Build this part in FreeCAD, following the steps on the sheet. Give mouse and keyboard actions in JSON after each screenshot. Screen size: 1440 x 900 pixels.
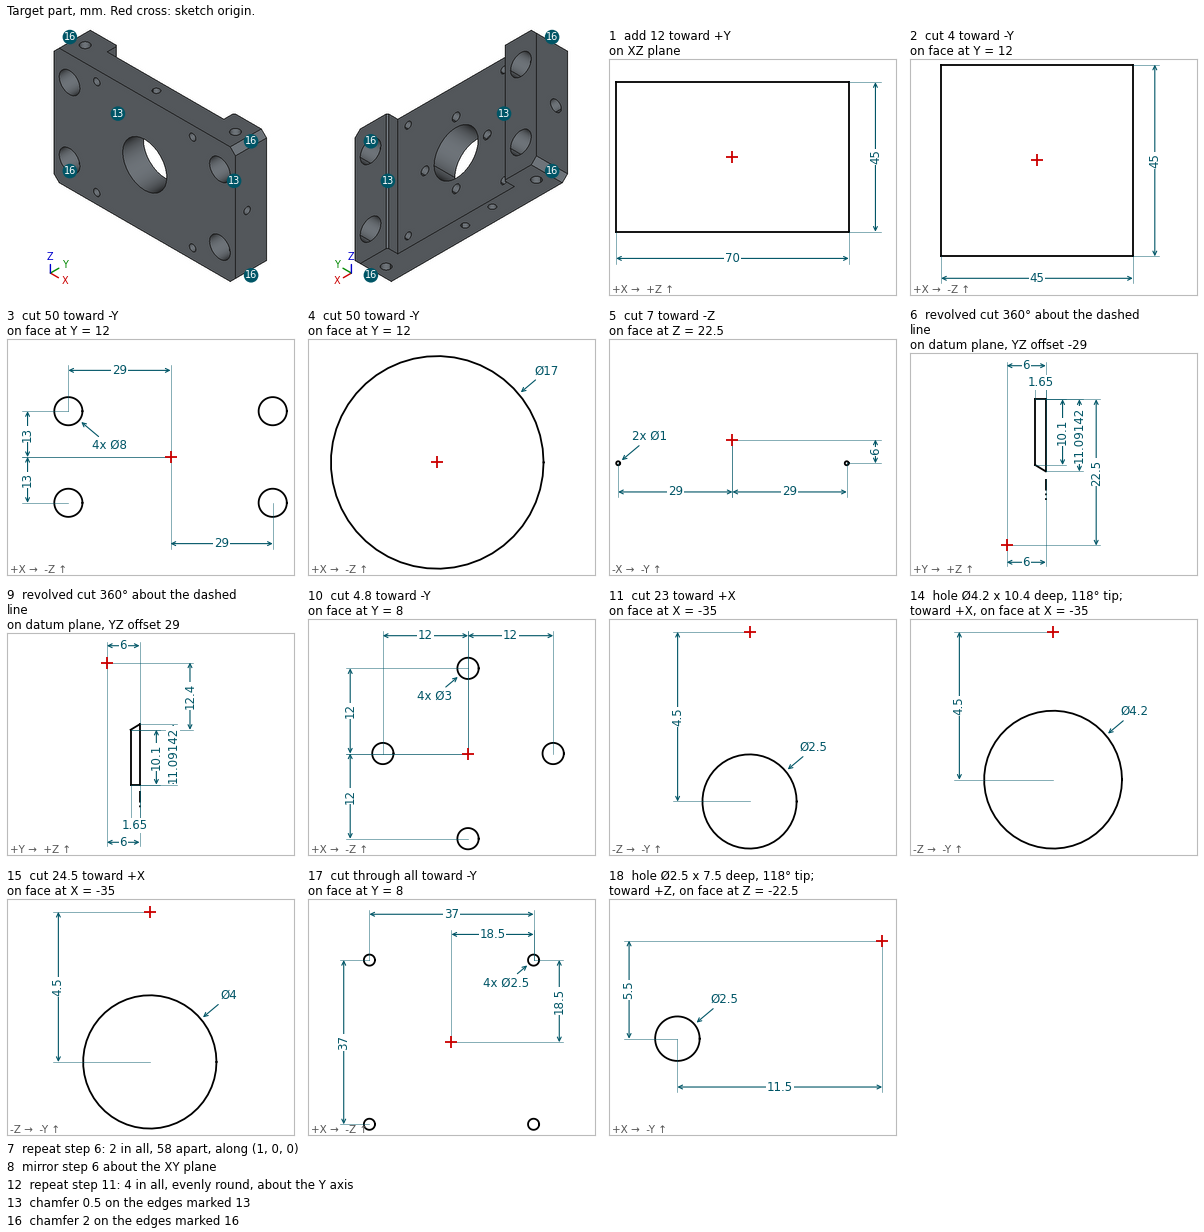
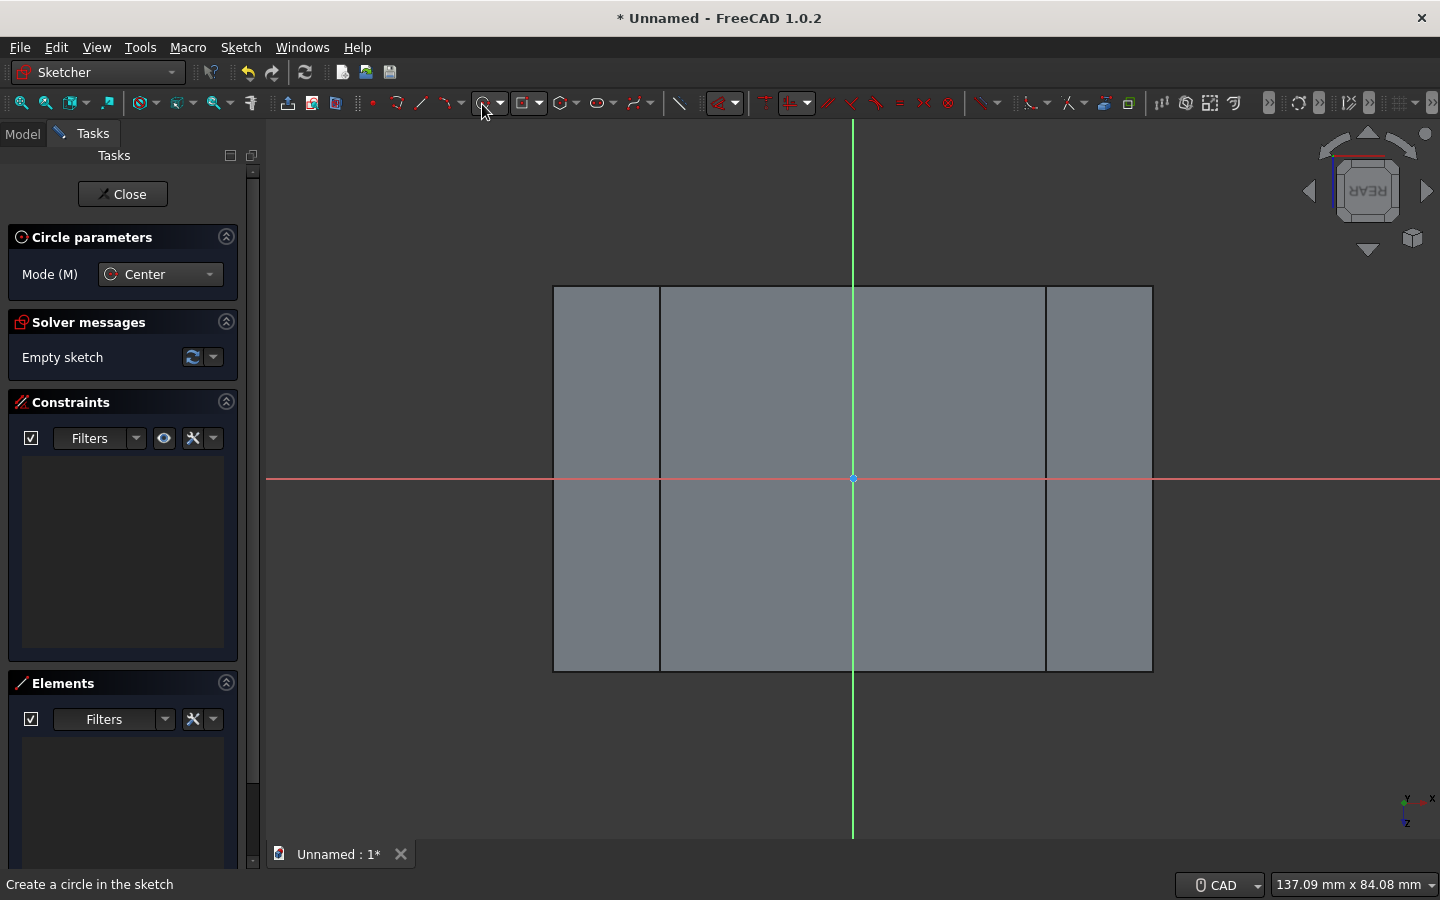
{"action": "left_click", "coordinate": [605, 368]}
{"action": "mouse_move", "coordinate": [629, 343]}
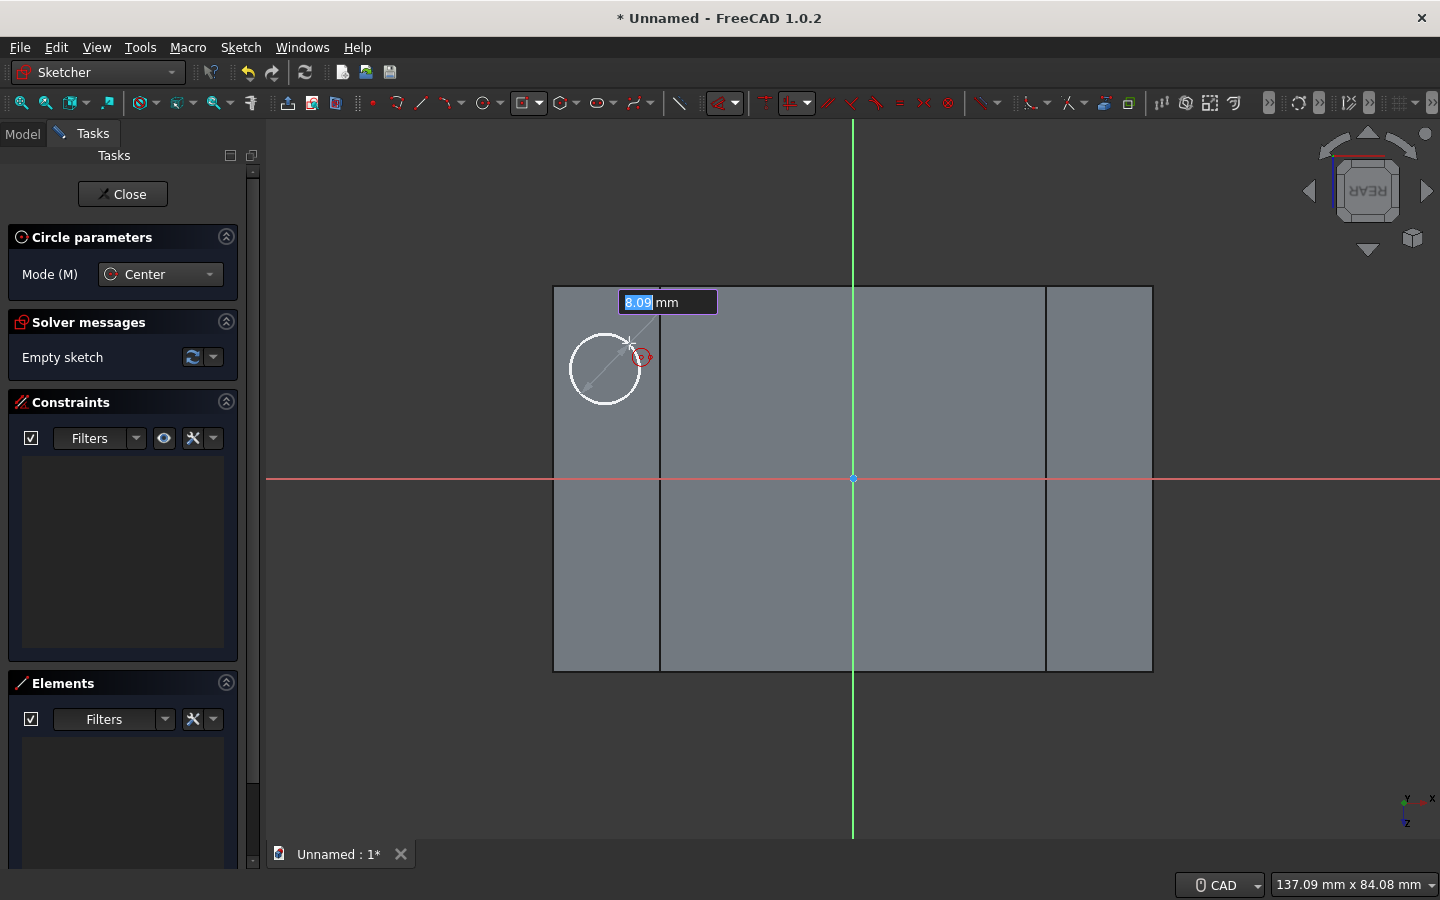
{"action": "type", "text": "8"}
{"action": "key", "text": "Return"}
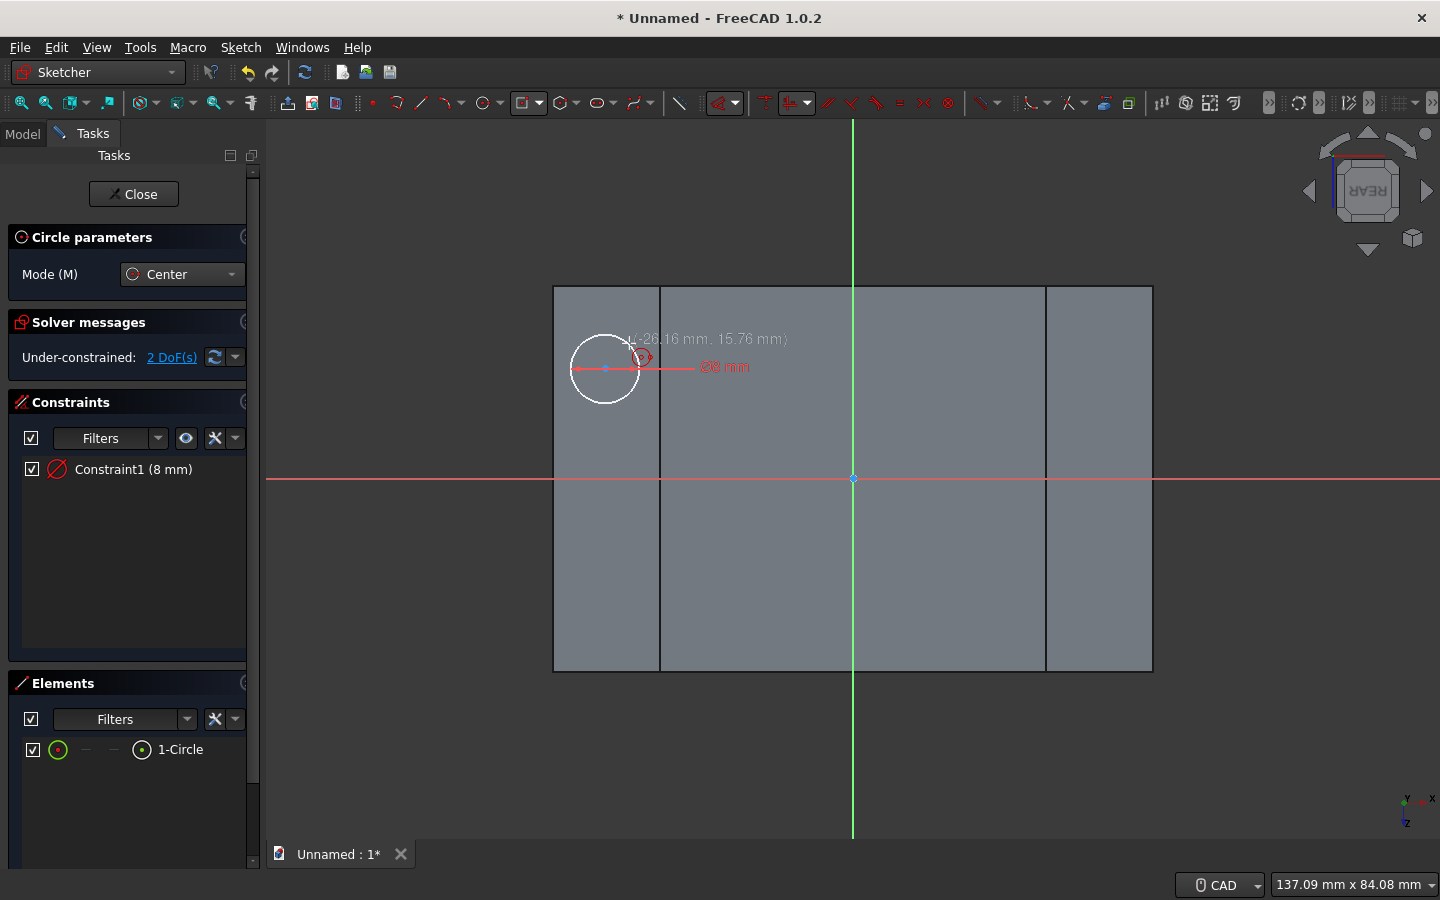
{"action": "left_click", "coordinate": [605, 590]}
{"action": "mouse_move", "coordinate": [629, 566]}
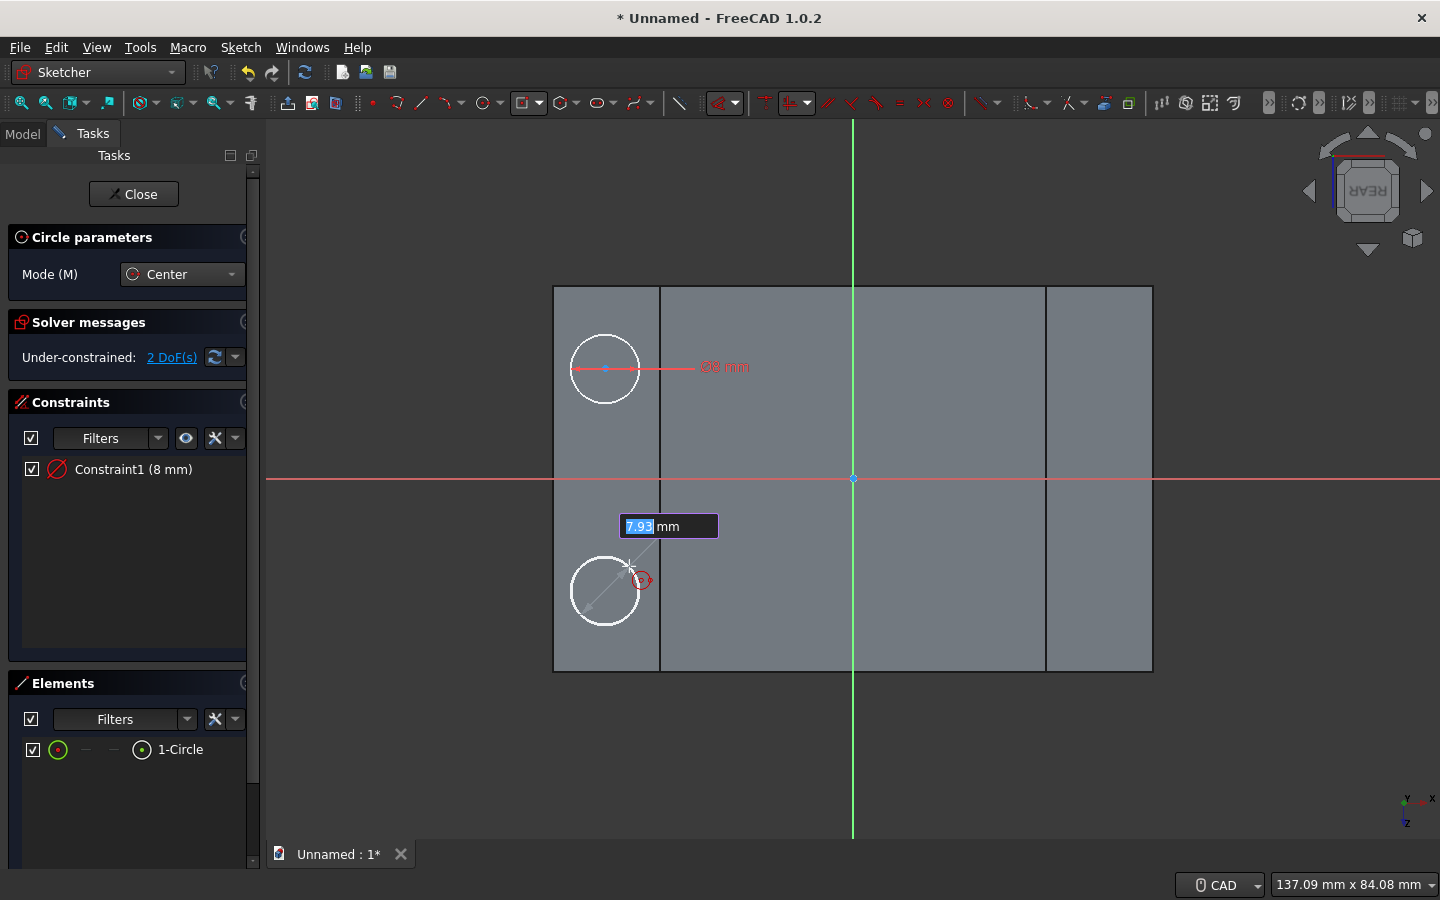
{"action": "type", "text": "8"}
{"action": "key", "text": "Return"}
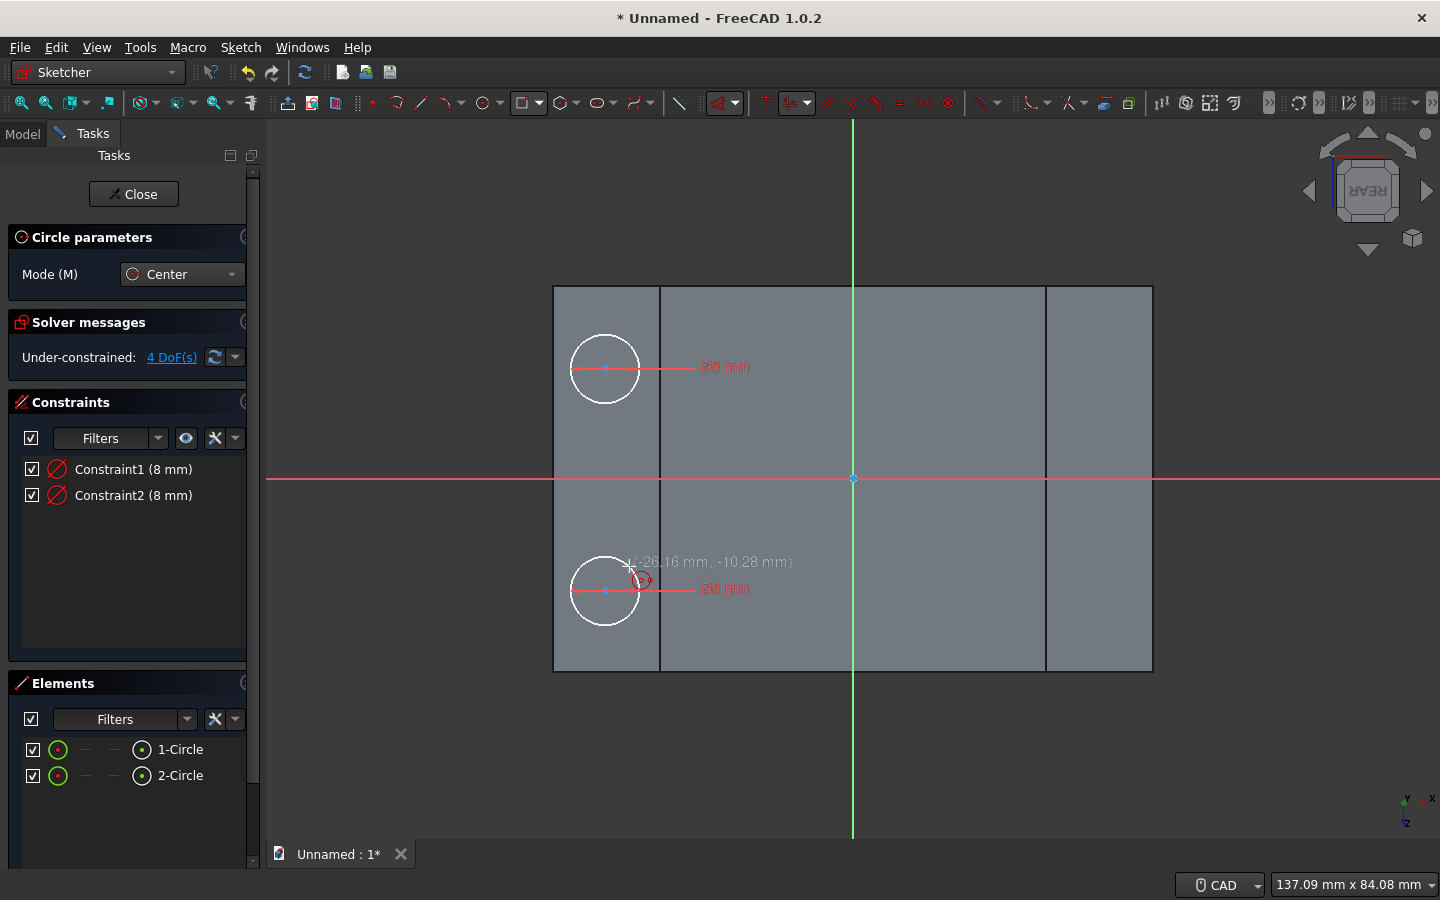
{"action": "left_click", "coordinate": [1101, 590]}
{"action": "mouse_move", "coordinate": [1126, 566]}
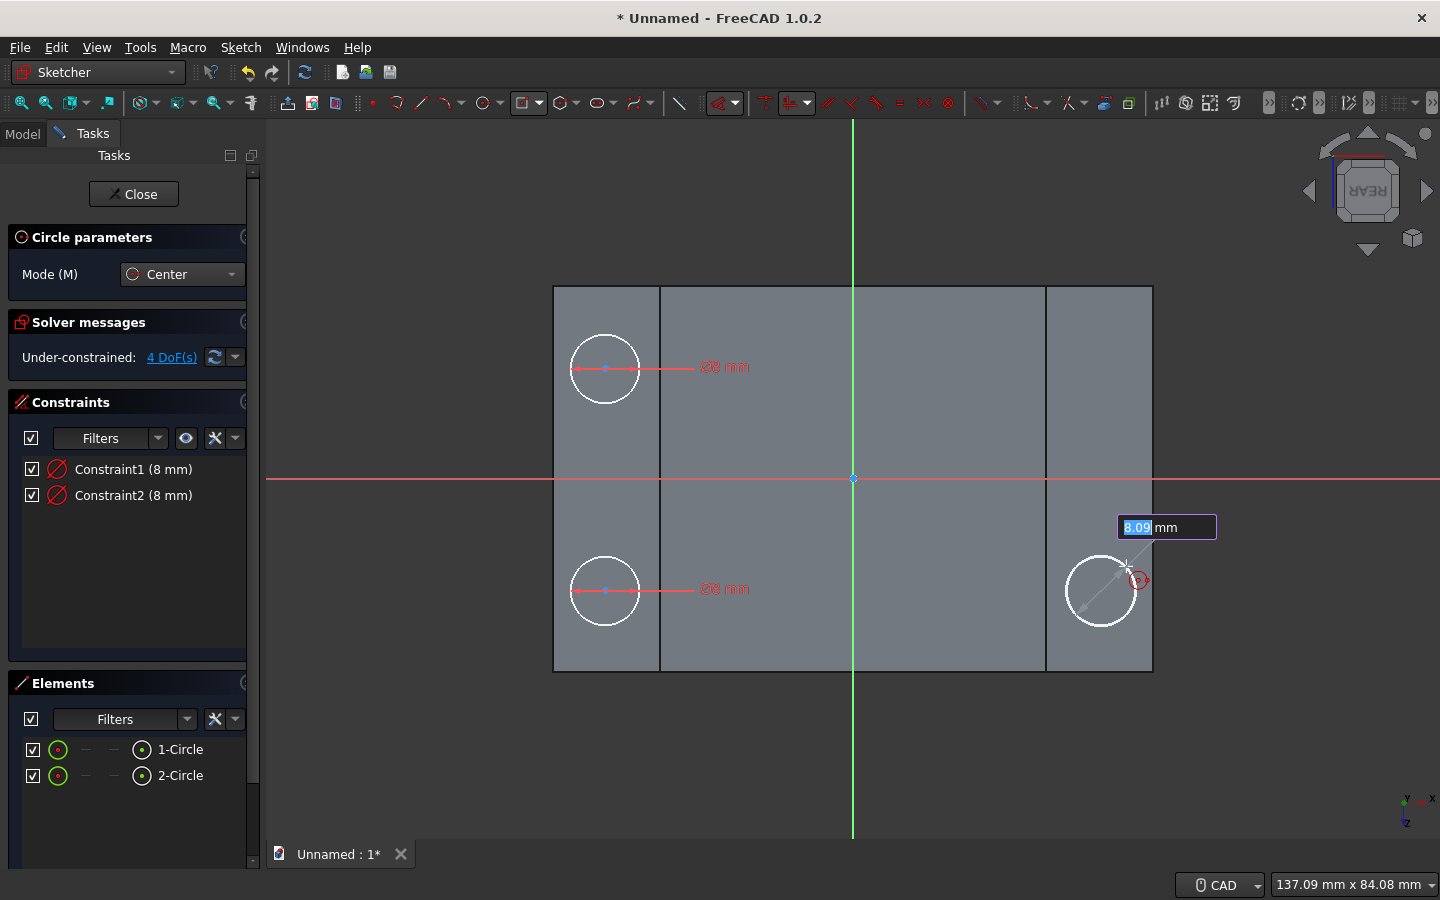
{"action": "type", "text": "8"}
{"action": "key", "text": "Return"}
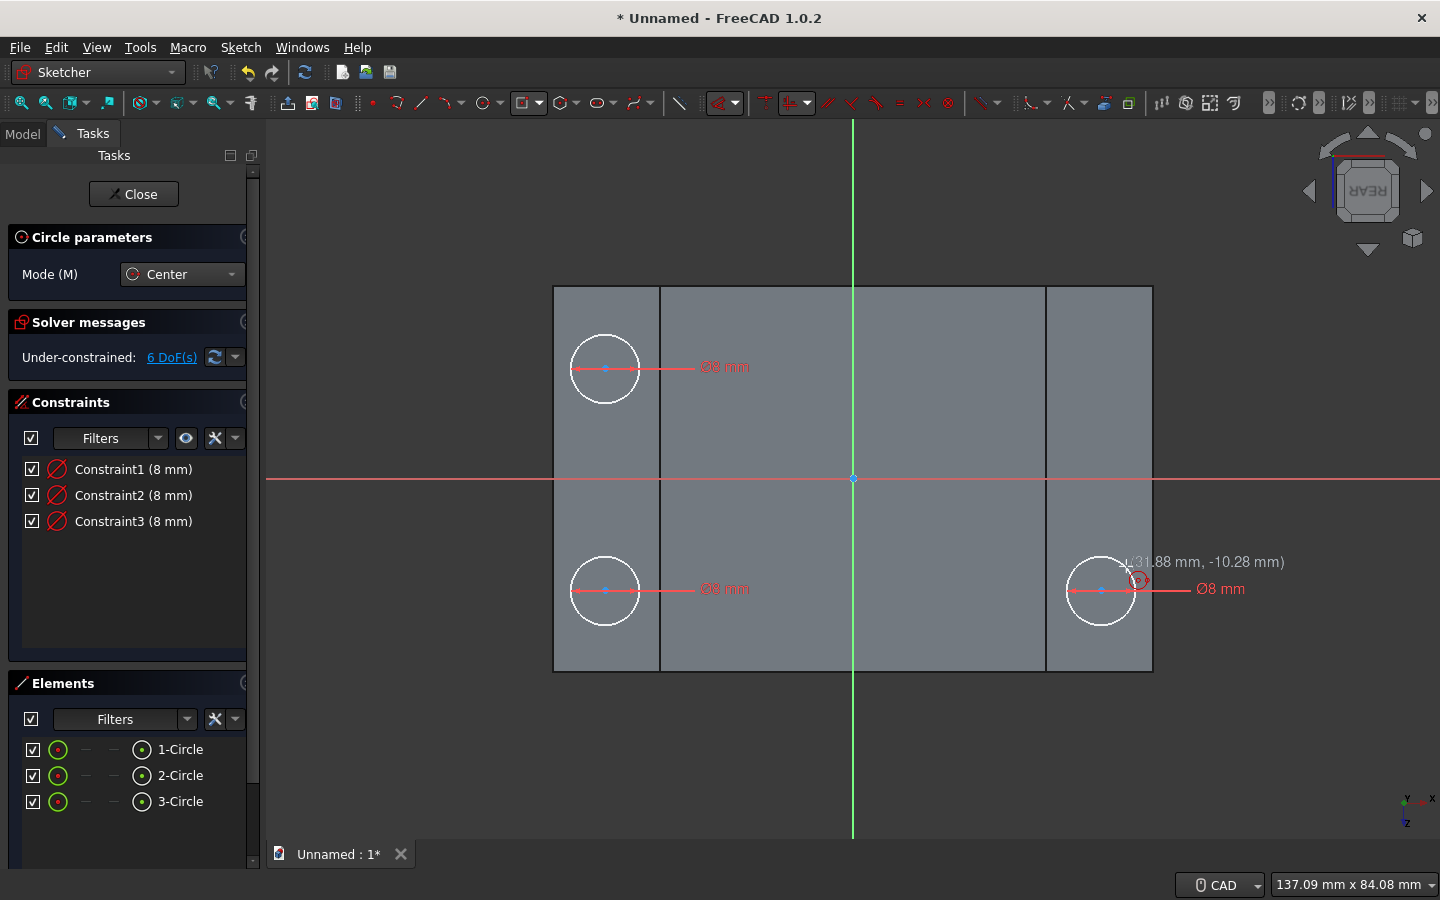
{"action": "left_click", "coordinate": [1101, 368]}
{"action": "mouse_move", "coordinate": [1126, 343]}